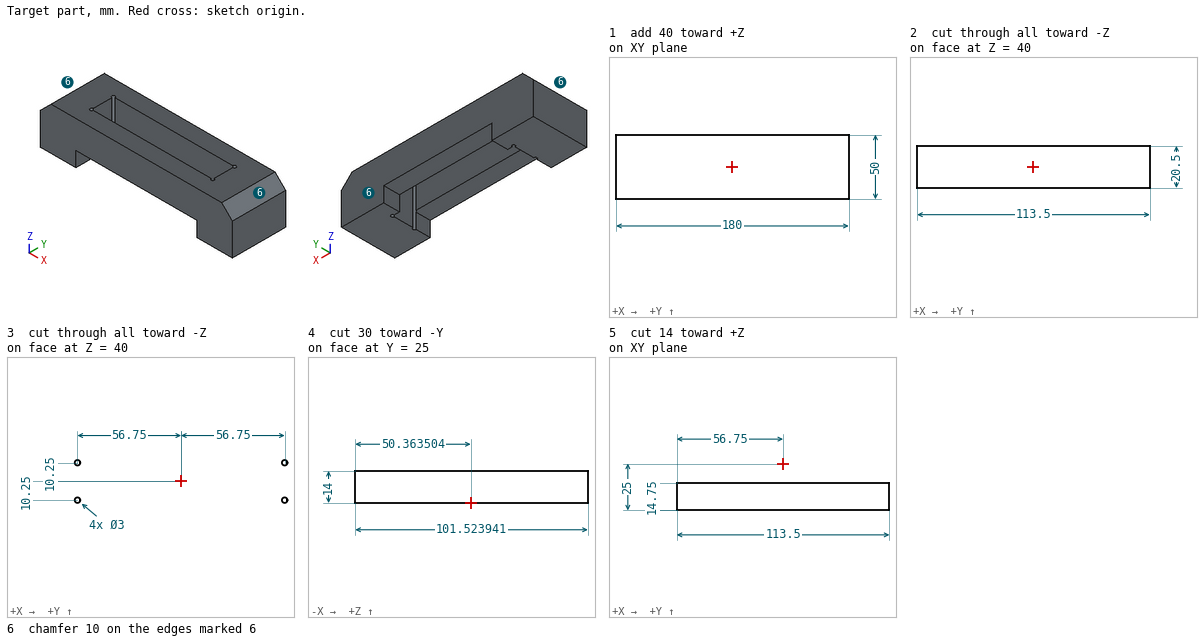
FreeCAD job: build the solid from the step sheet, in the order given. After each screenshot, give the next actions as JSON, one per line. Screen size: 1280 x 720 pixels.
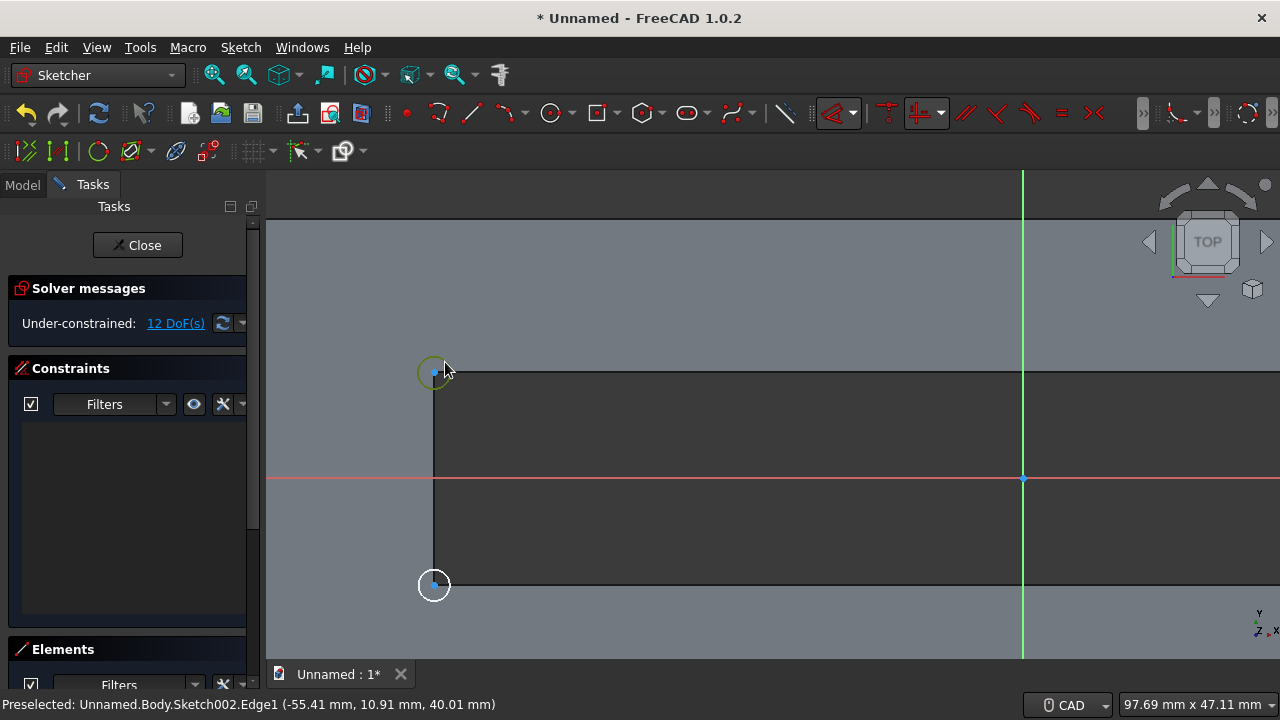
{"action": "left_click", "coordinate": [445, 574]}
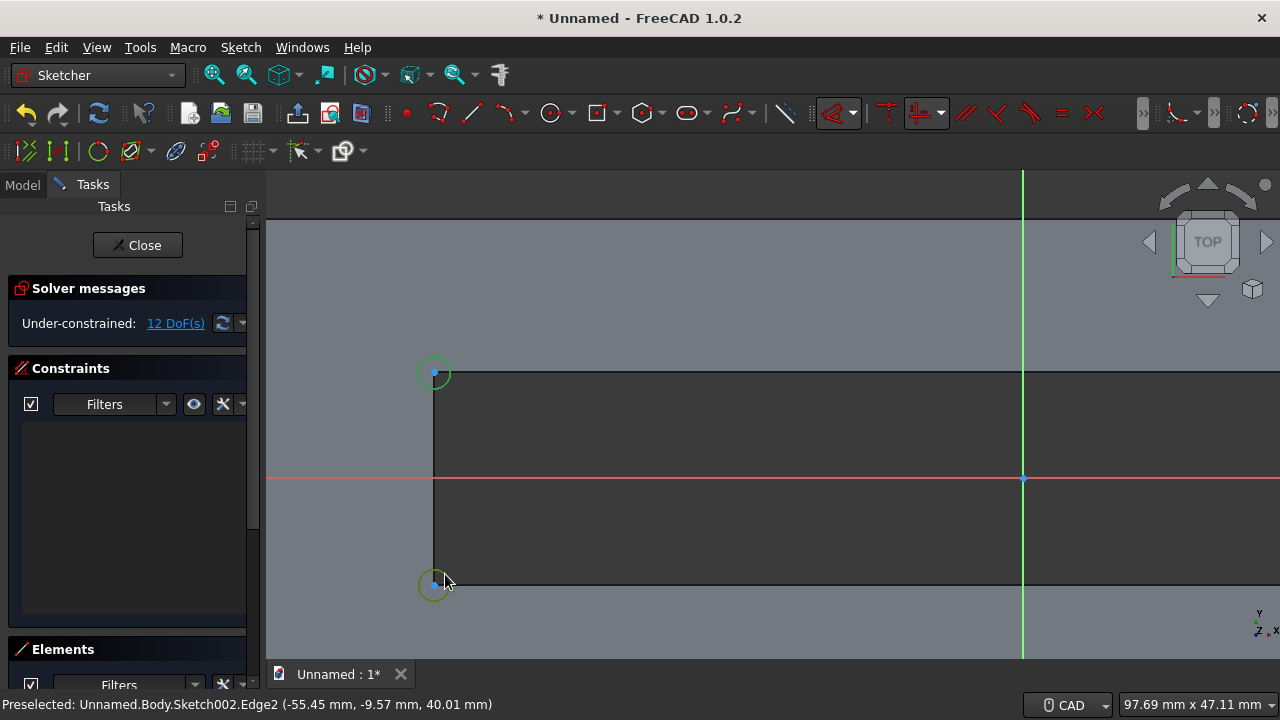
{"action": "scroll", "coordinate": [444, 362], "scroll_direction": "down", "scroll_amount": 4}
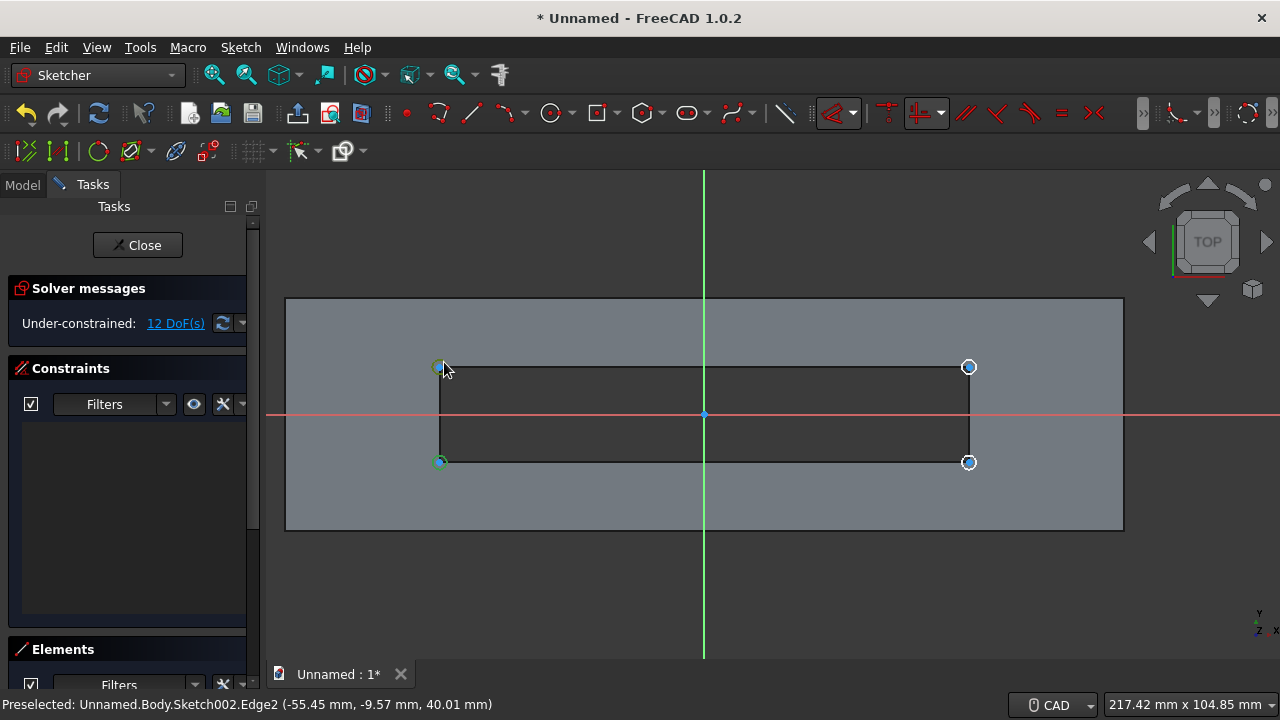
{"action": "scroll", "coordinate": [974, 362], "scroll_direction": "up", "scroll_amount": 4}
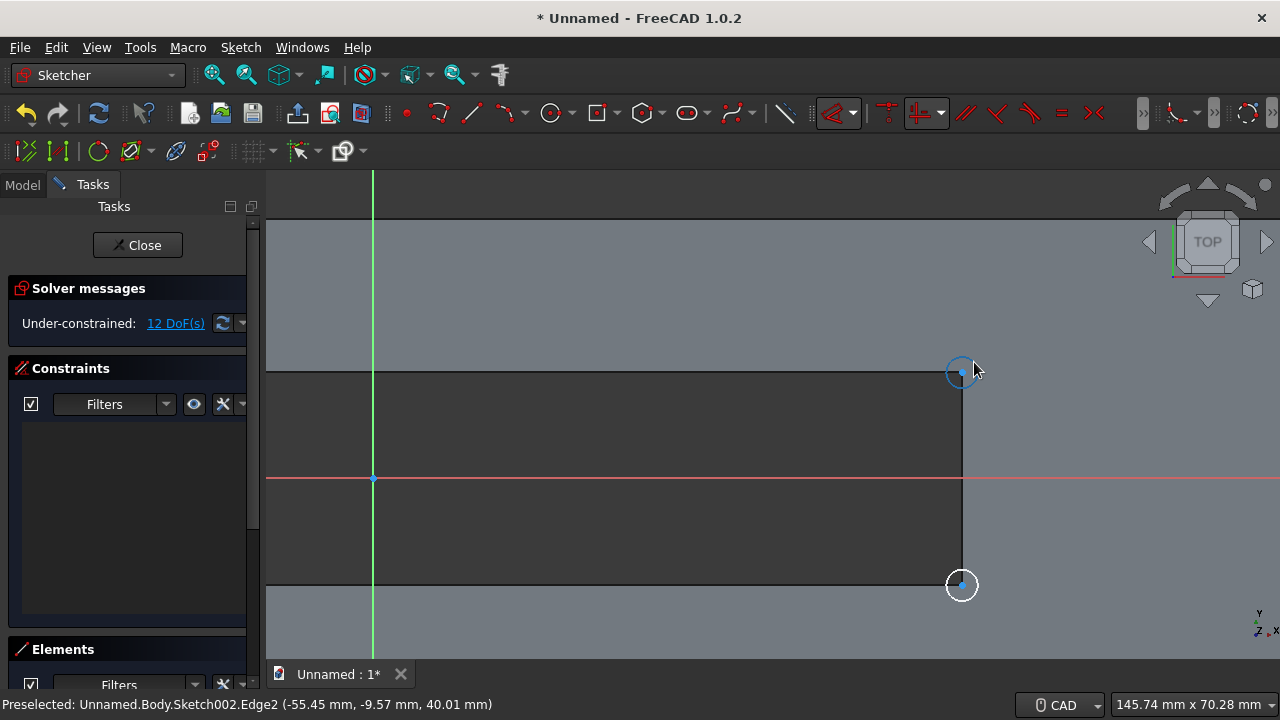
{"action": "left_click", "coordinate": [973, 362]}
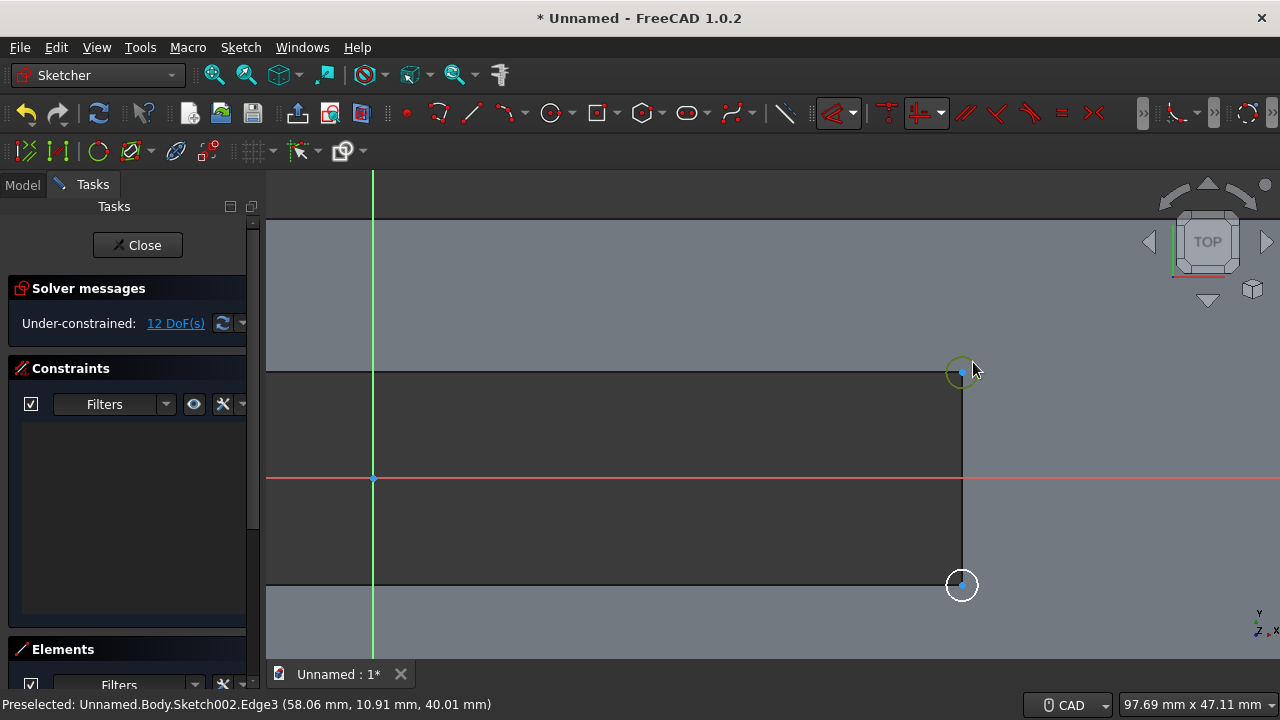
{"action": "left_click", "coordinate": [973, 574]}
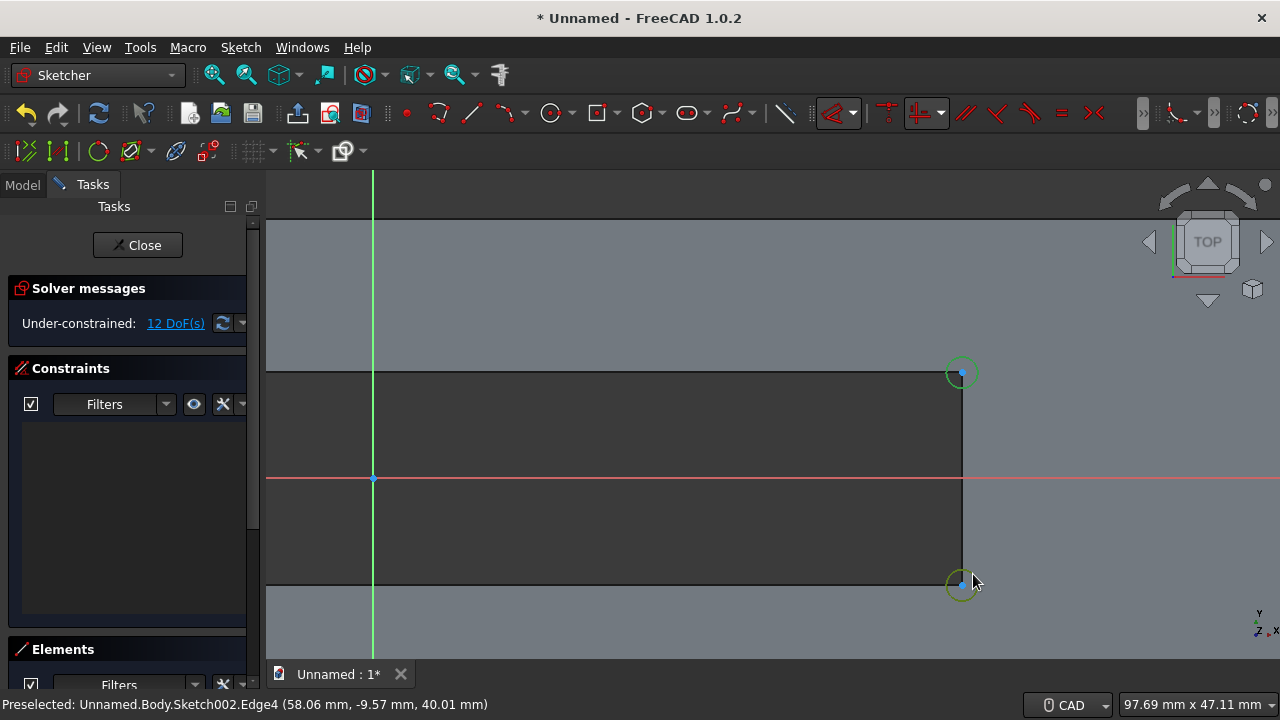
{"action": "left_click", "coordinate": [1062, 114]}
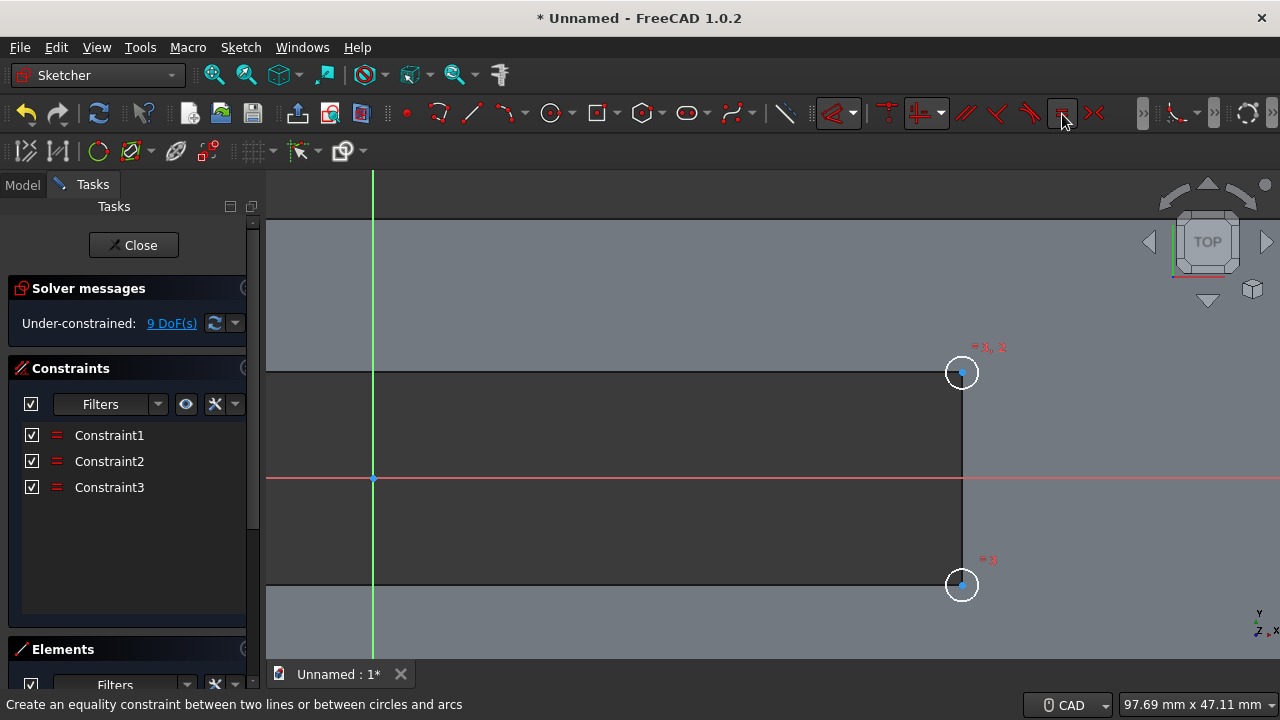
{"action": "scroll", "coordinate": [975, 362], "scroll_direction": "down", "scroll_amount": 4}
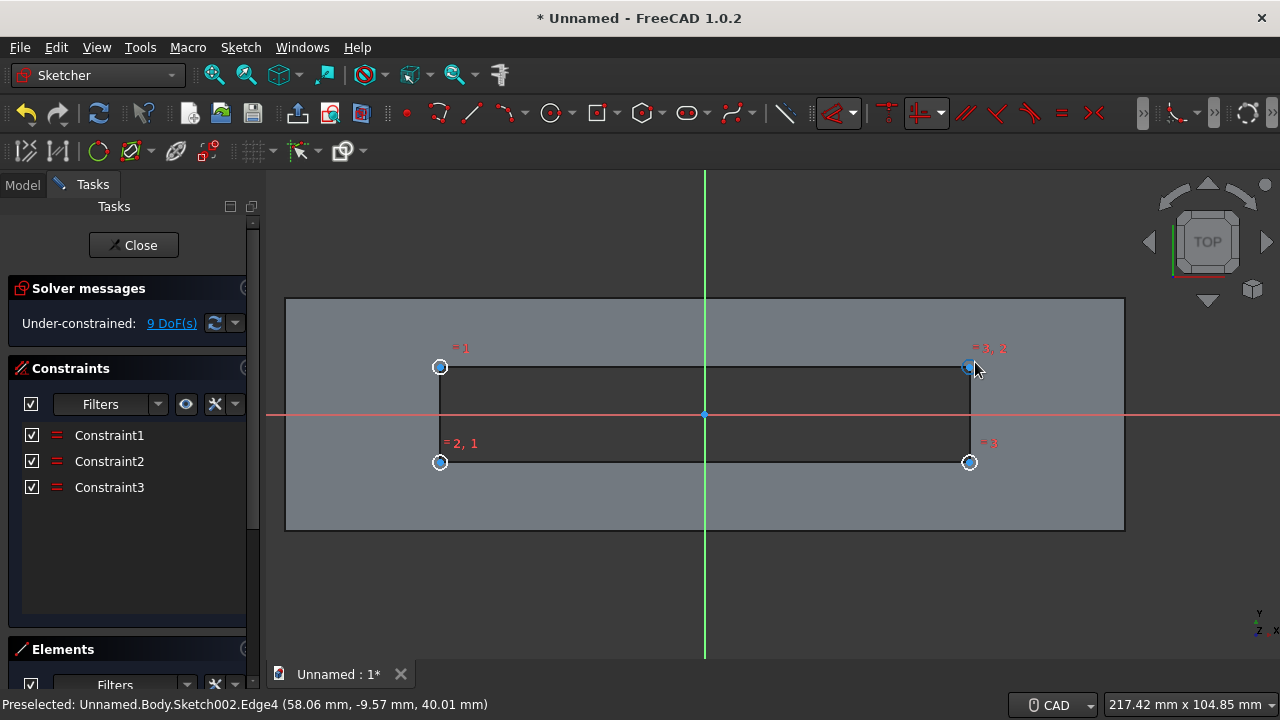
{"action": "left_click", "coordinate": [440, 367]}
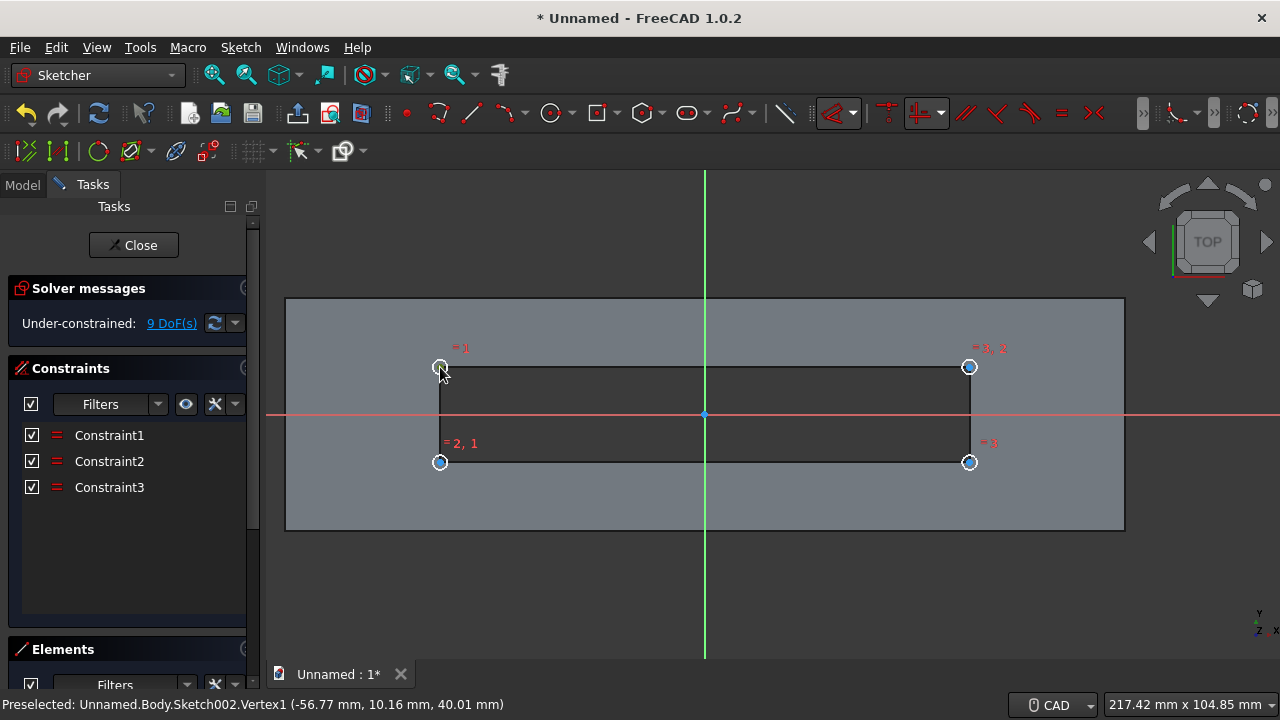
{"action": "left_click", "coordinate": [440, 463]}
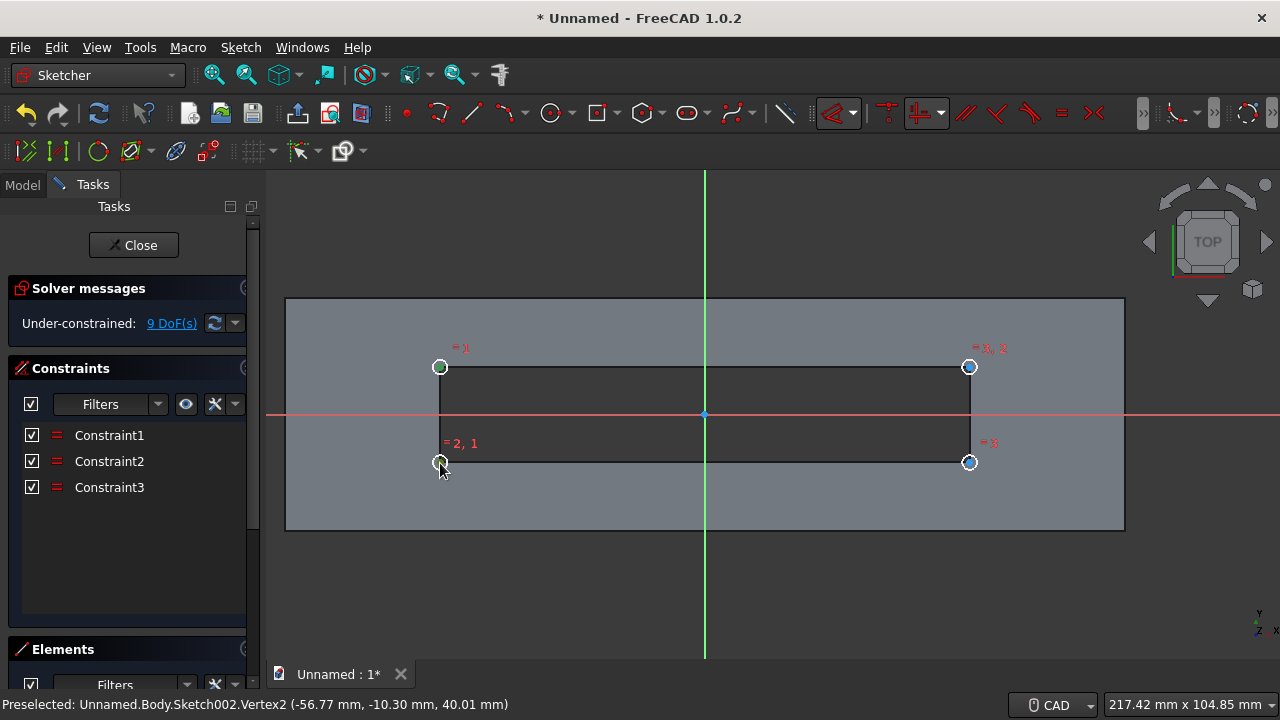
{"action": "key", "text": "v"}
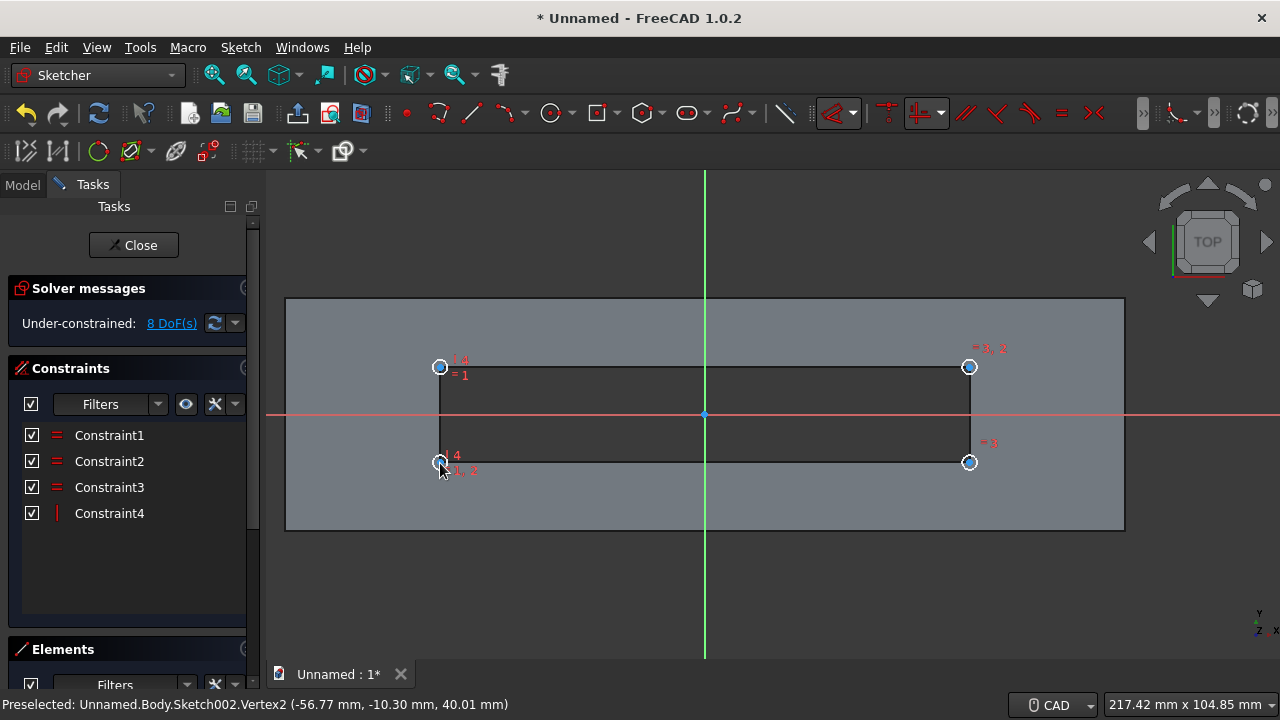
{"action": "left_click", "coordinate": [440, 367]}